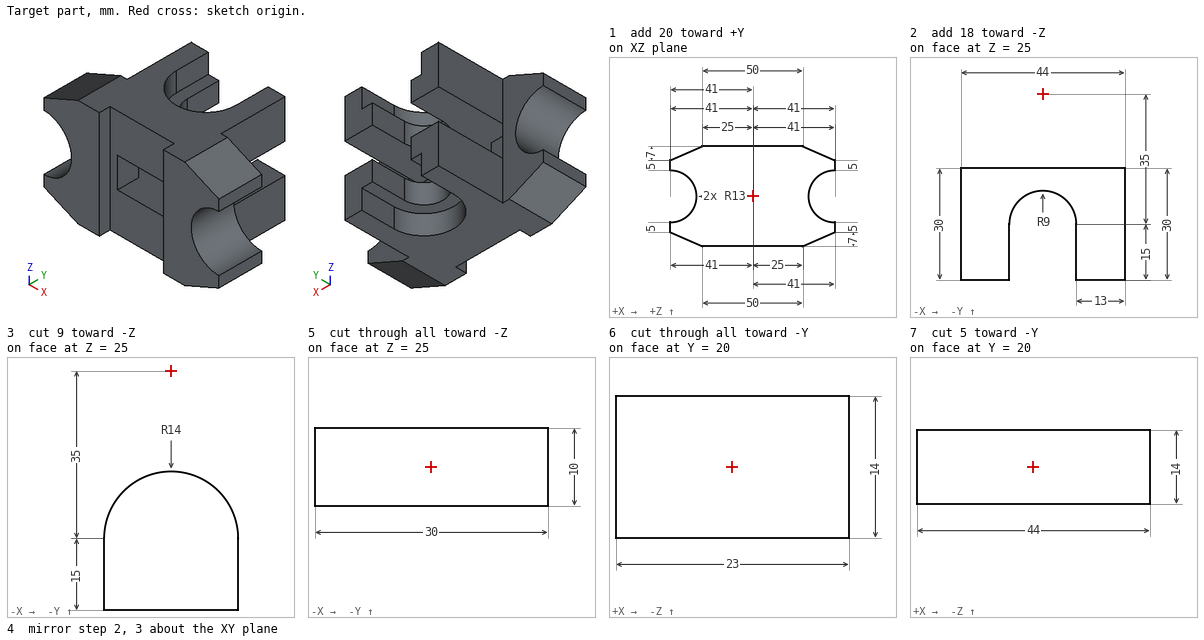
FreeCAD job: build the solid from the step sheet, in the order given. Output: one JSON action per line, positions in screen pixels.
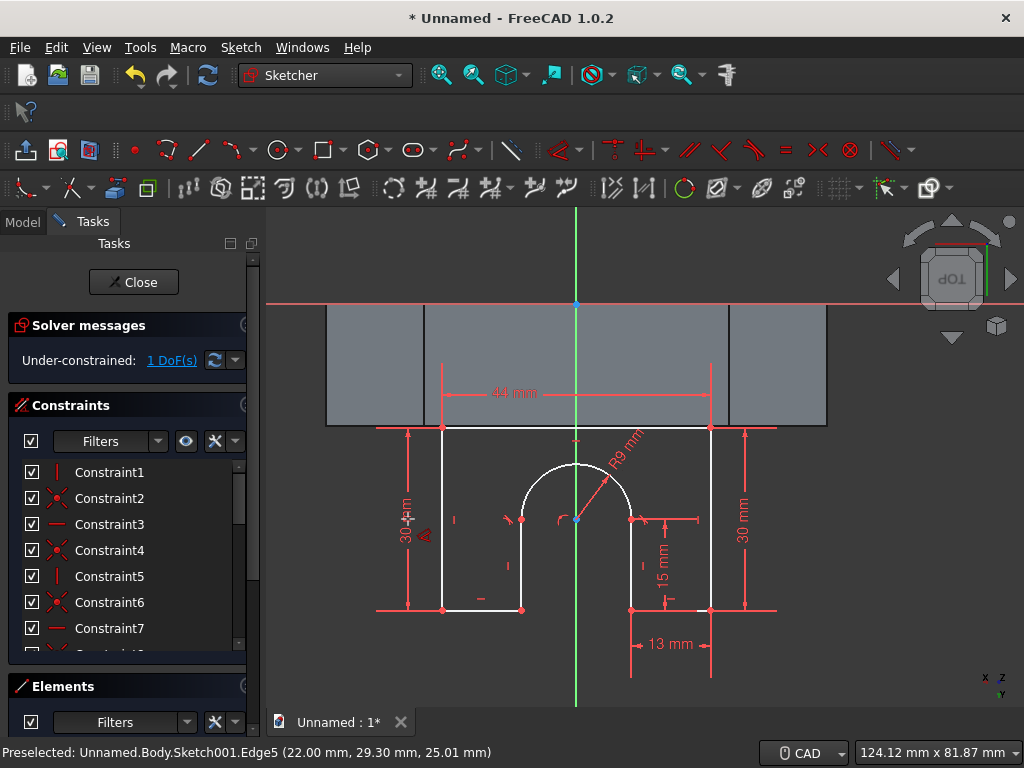
{"action": "left_click", "coordinate": [631, 519]}
{"action": "left_click", "coordinate": [665, 412]}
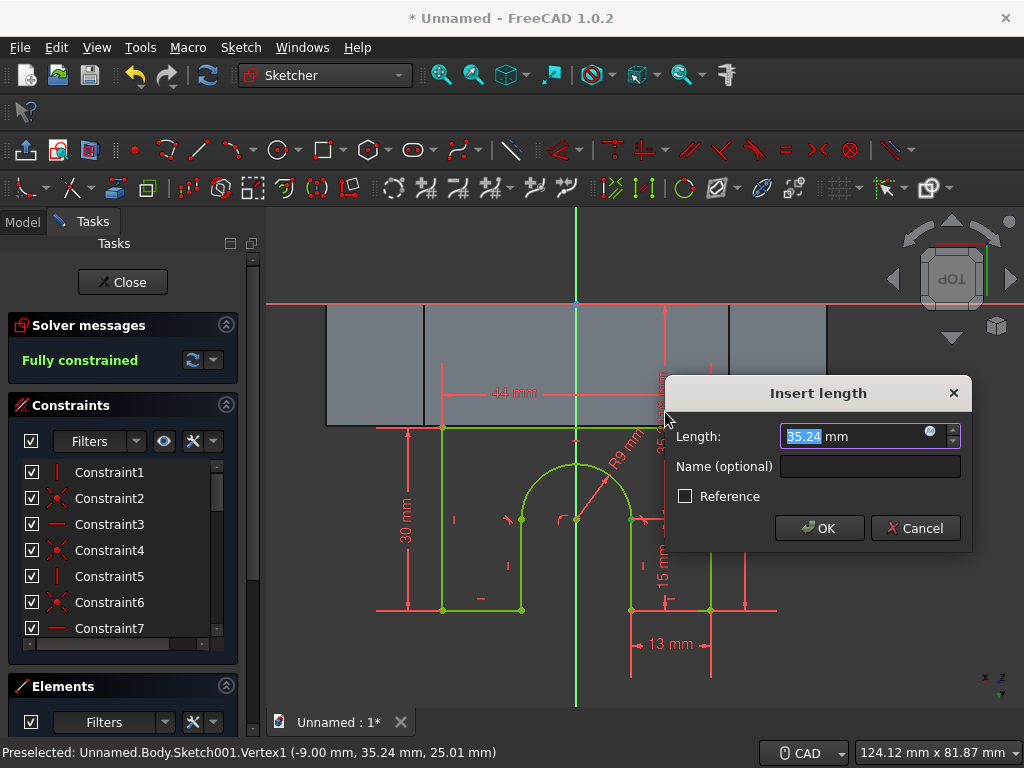
{"action": "type", "text": "35"}
{"action": "key", "text": "Return"}
{"action": "key", "text": "Escape"}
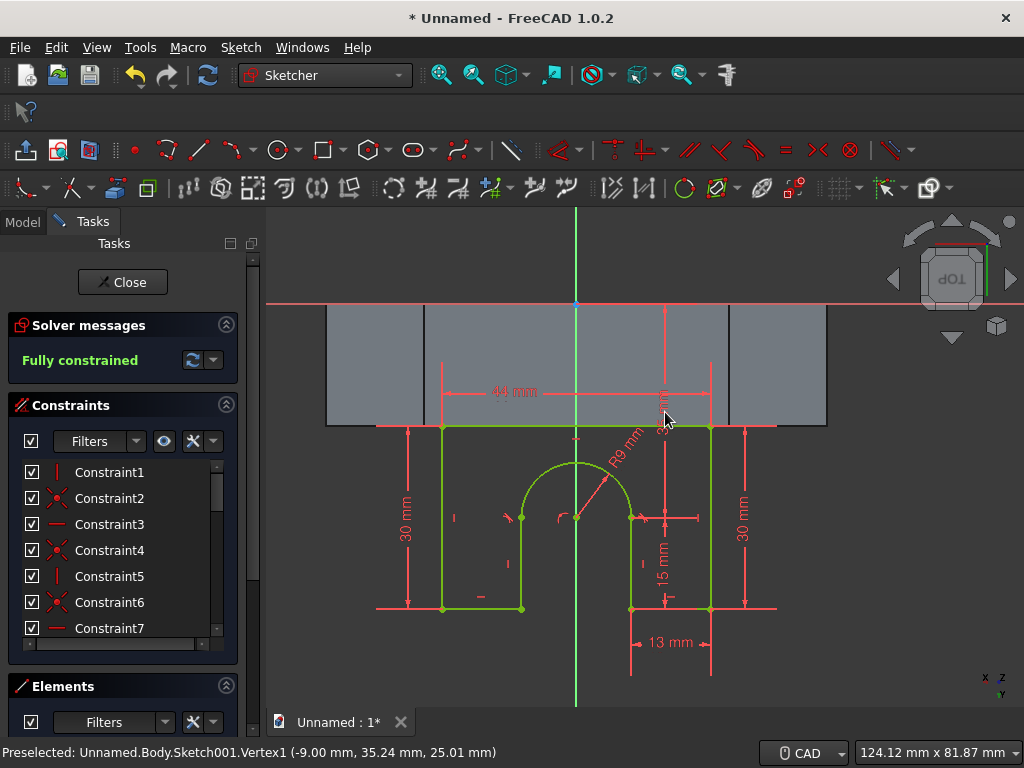
{"action": "left_click", "coordinate": [123, 282]}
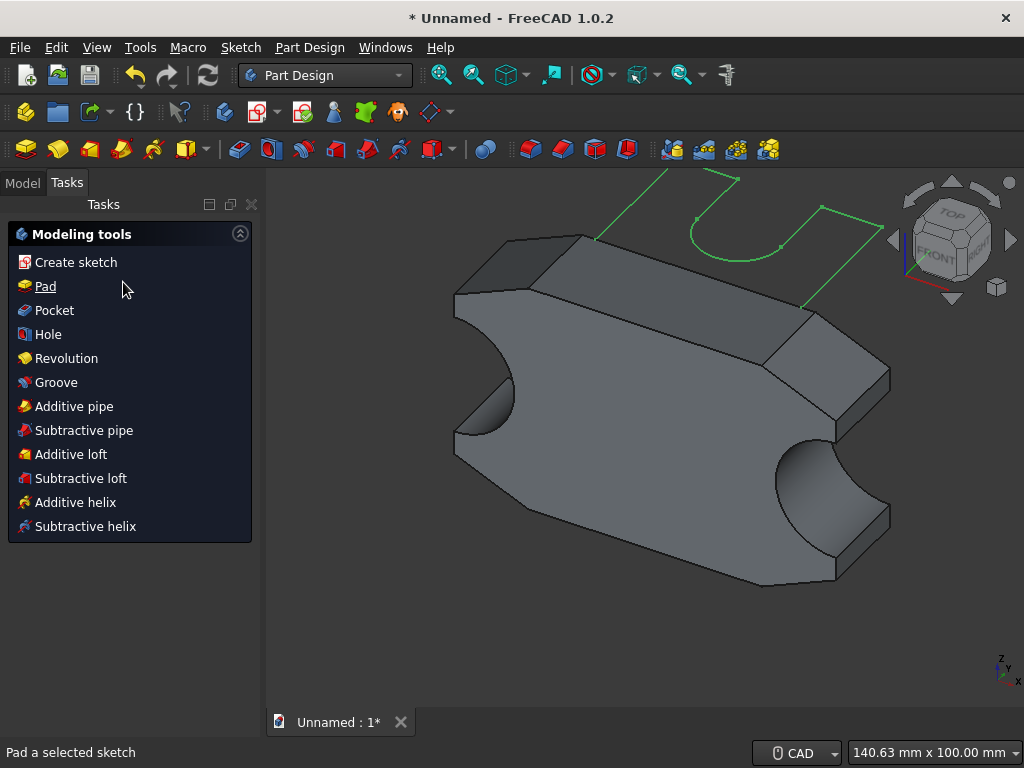
{"action": "left_click", "coordinate": [26, 150]}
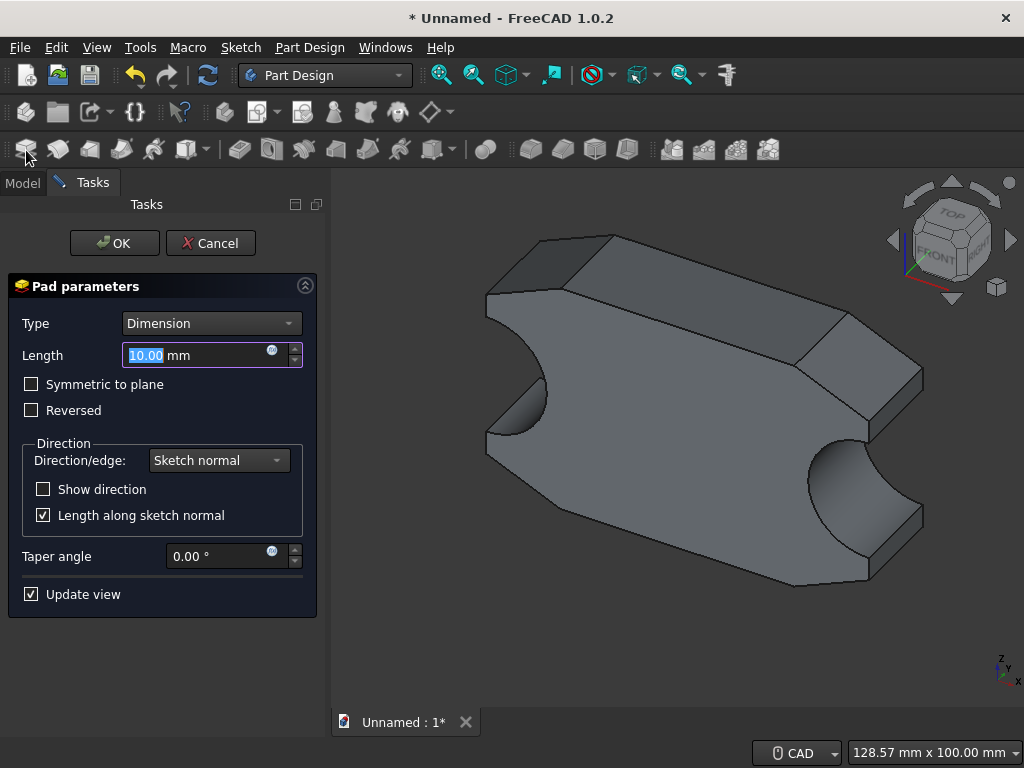
{"action": "type", "text": "18"}
{"action": "key", "text": "Tab"}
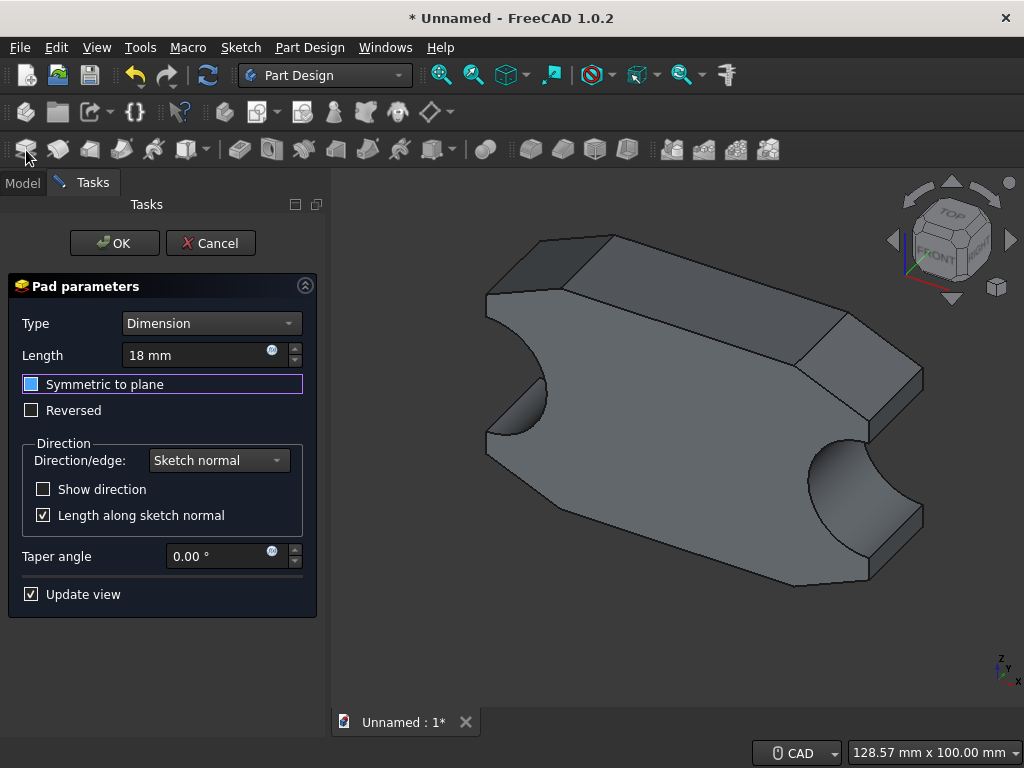
{"action": "left_click", "coordinate": [30, 410]}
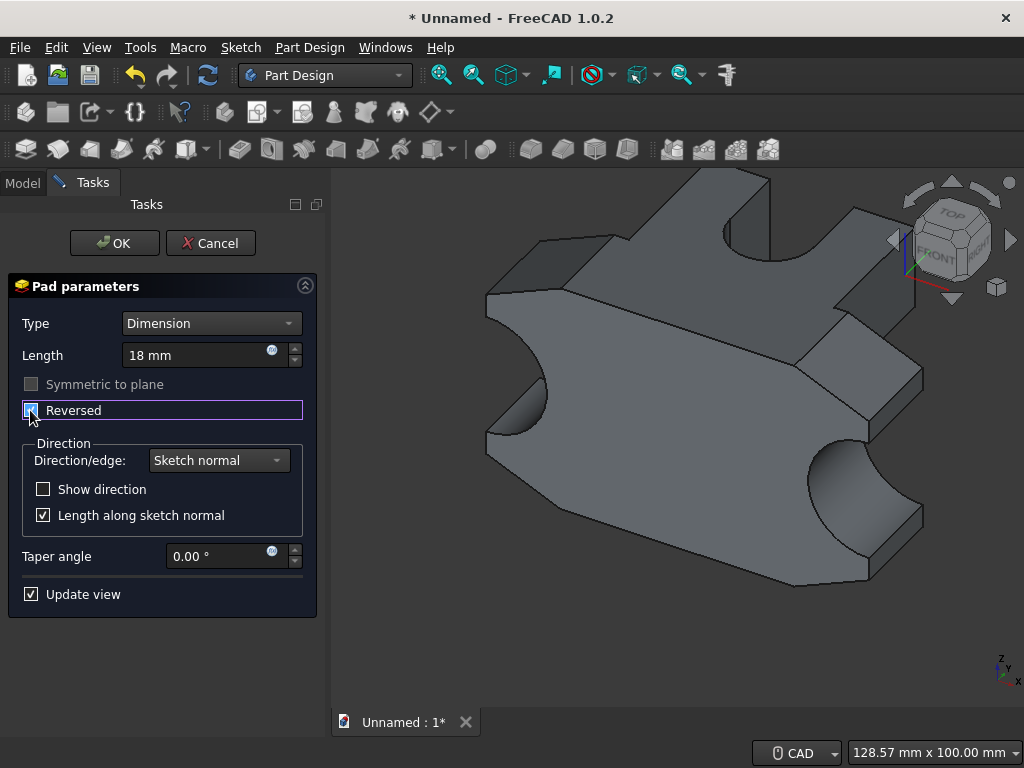
{"action": "left_click", "coordinate": [115, 243]}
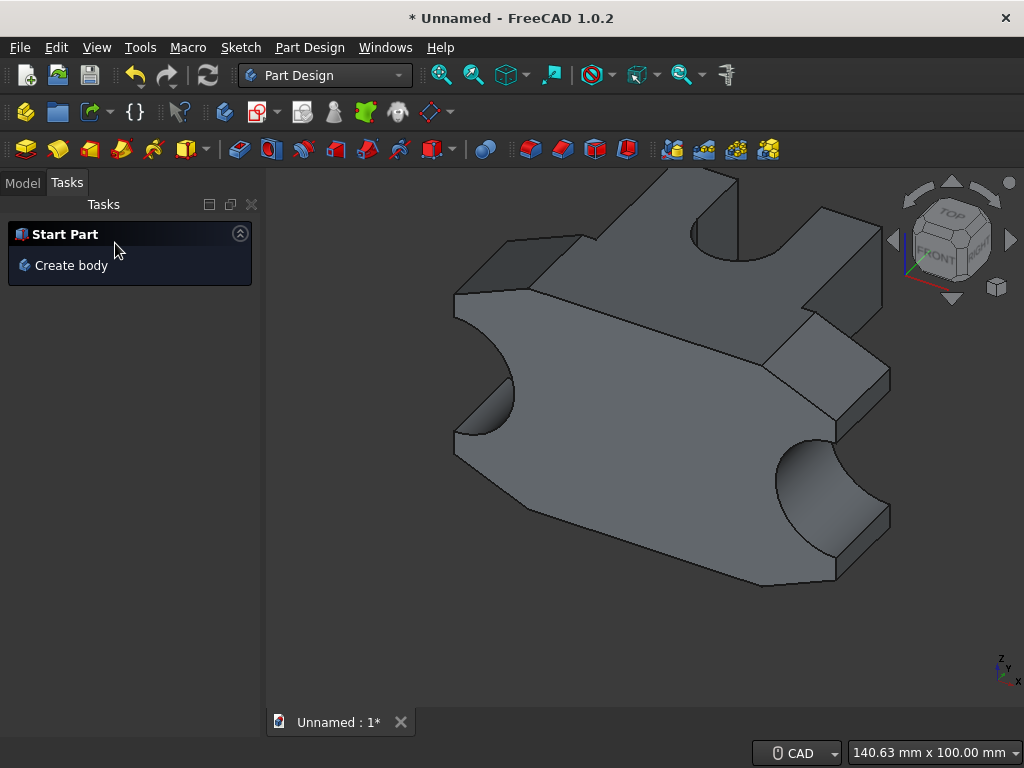
{"action": "left_click", "coordinate": [442, 76]}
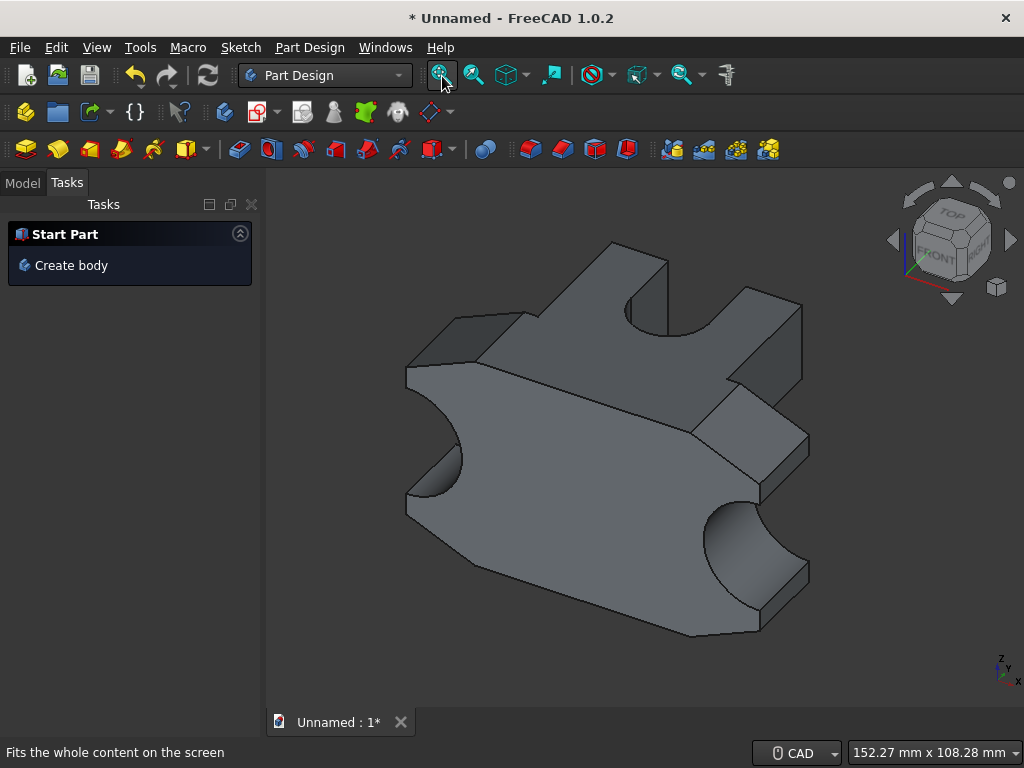
{"action": "left_click", "coordinate": [671, 390]}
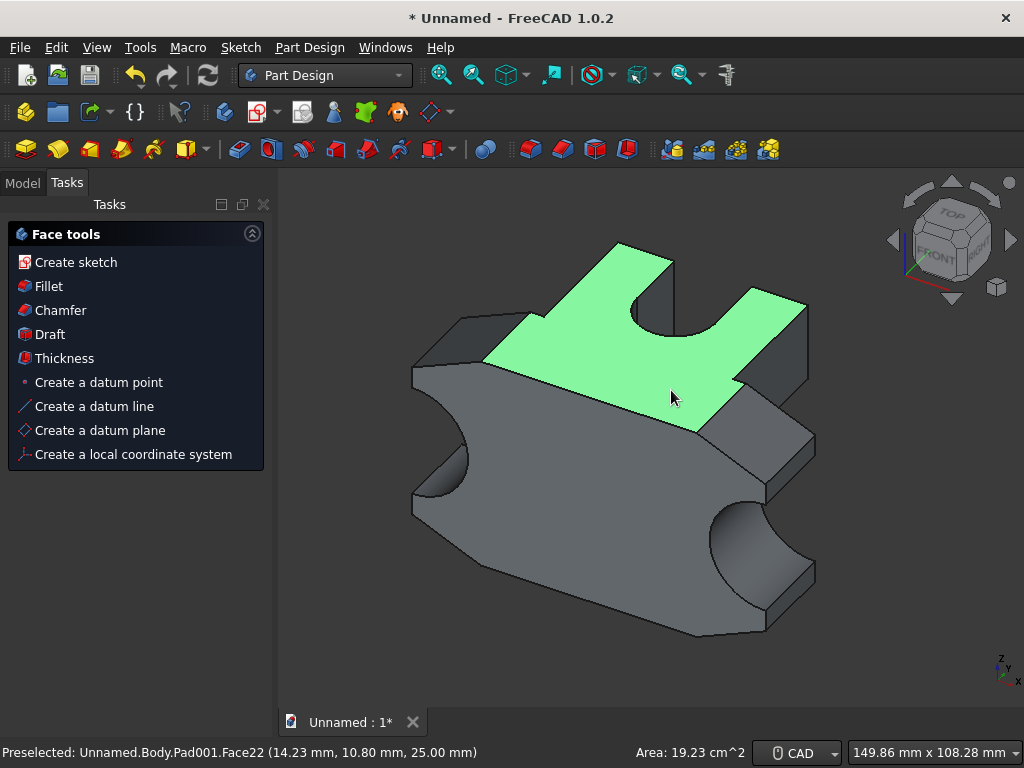
{"action": "left_click", "coordinate": [258, 112]}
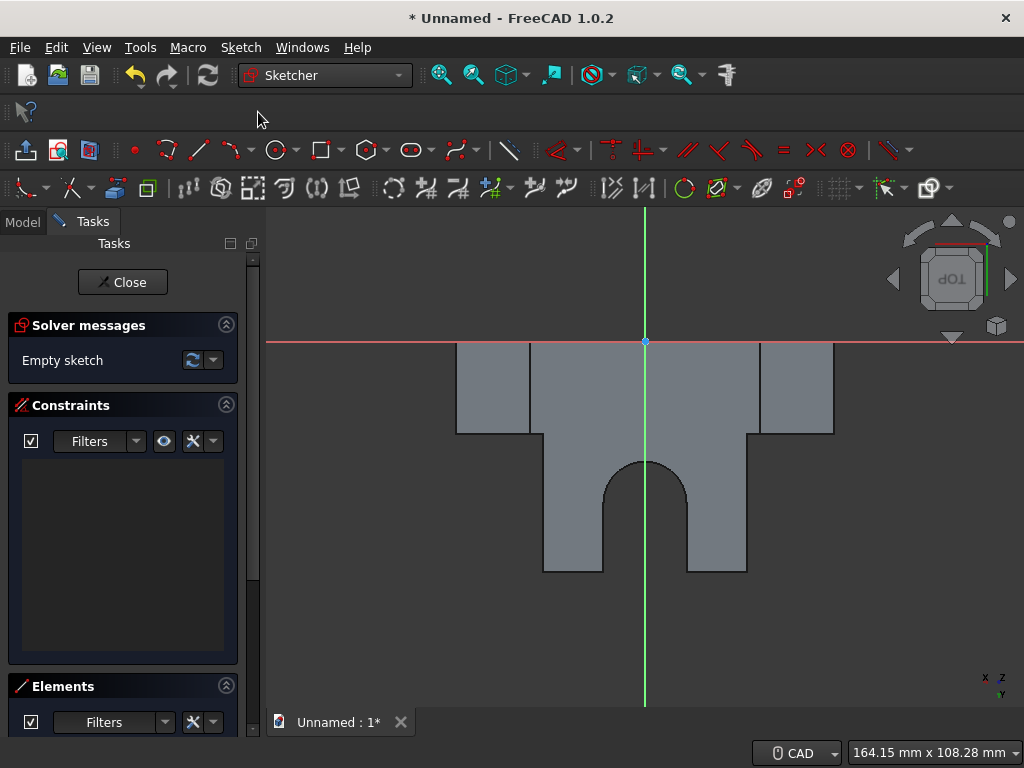
{"action": "scroll", "coordinate": [784, 457], "scroll_direction": "up", "scroll_amount": 2}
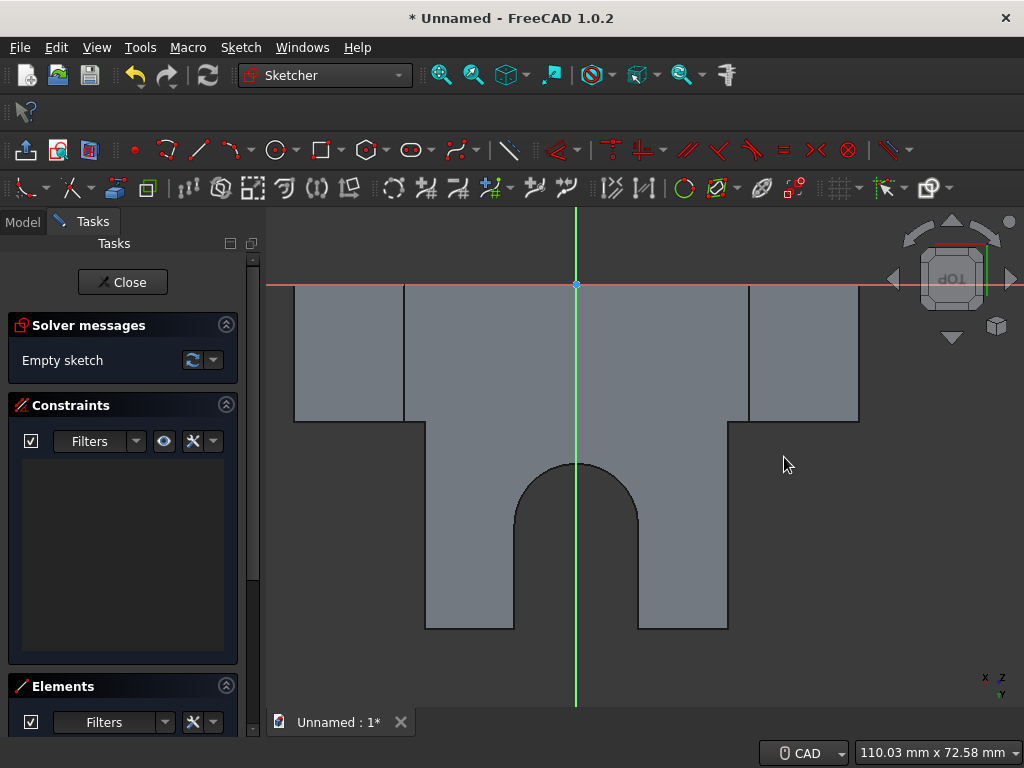
{"action": "left_click", "coordinate": [168, 150]}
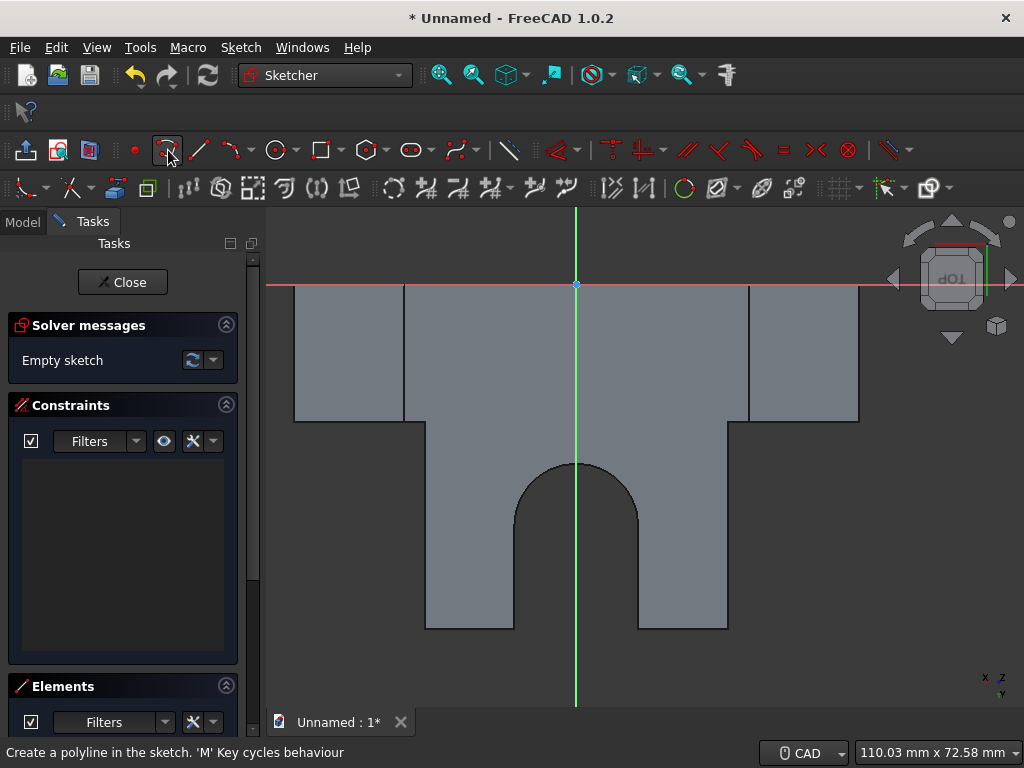
{"action": "left_click", "coordinate": [480, 526]}
{"action": "left_click", "coordinate": [480, 629]}
{"action": "left_click", "coordinate": [673, 629]}
{"action": "left_click", "coordinate": [673, 526]}
{"action": "right_click", "coordinate": [673, 526]}